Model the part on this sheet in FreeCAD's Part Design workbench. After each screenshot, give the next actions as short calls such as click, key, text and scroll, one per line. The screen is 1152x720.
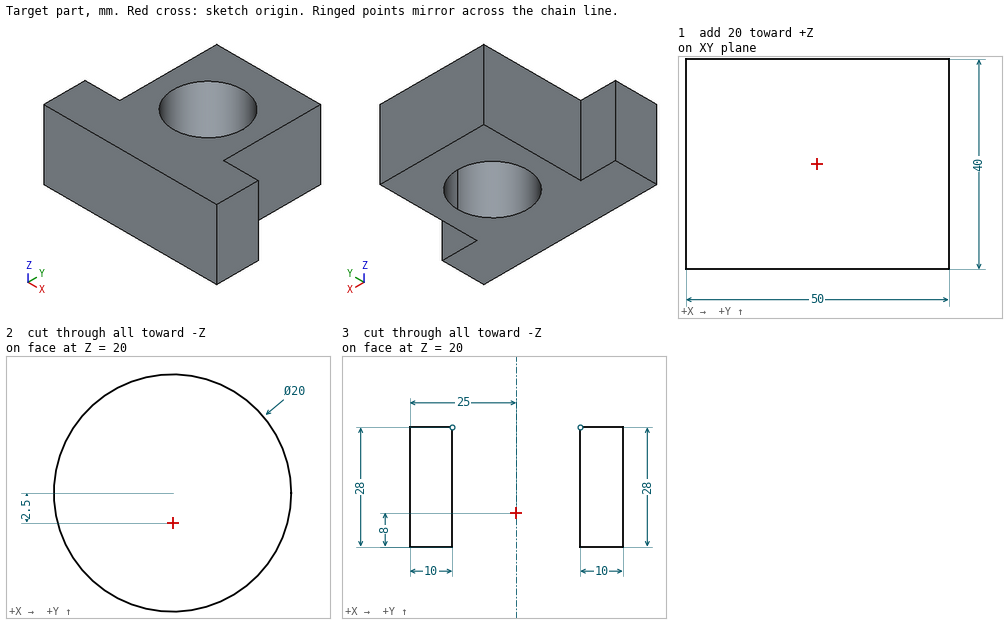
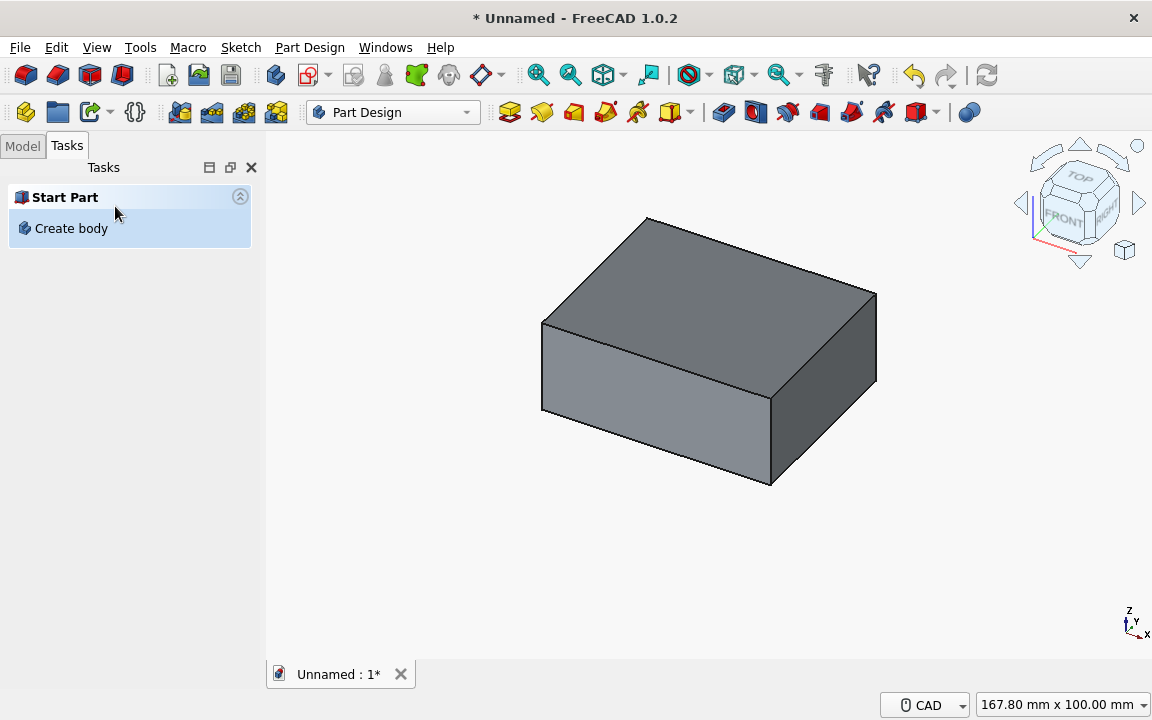
click(709, 307)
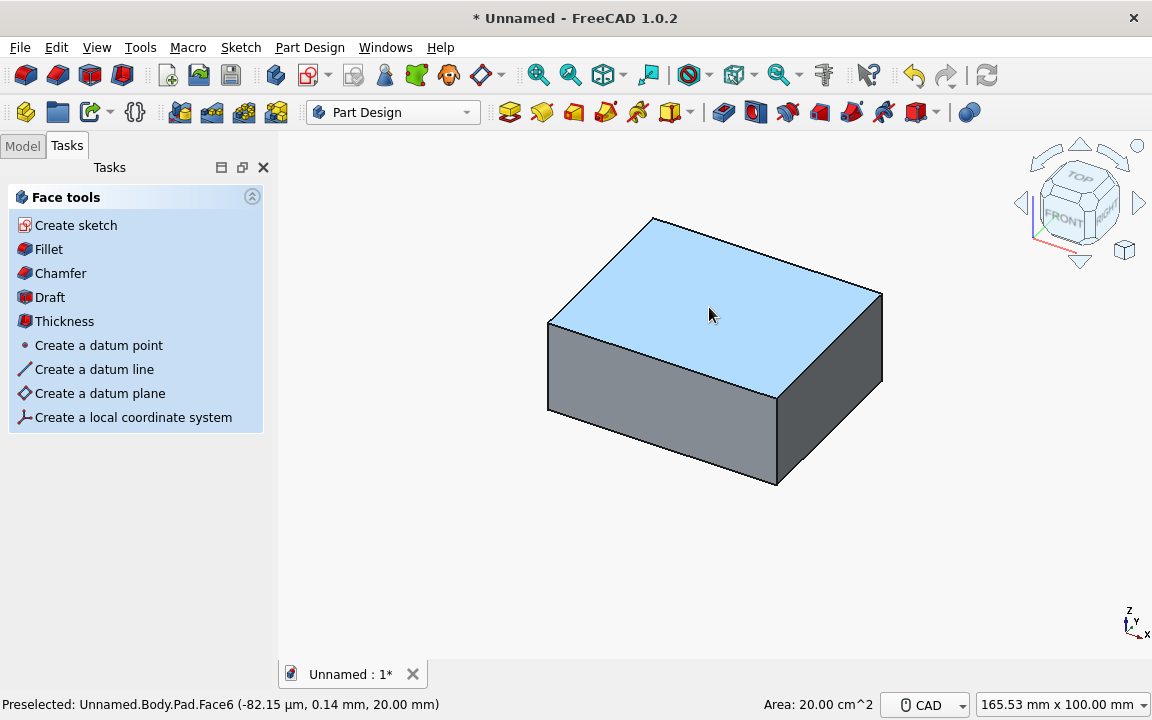
click(308, 76)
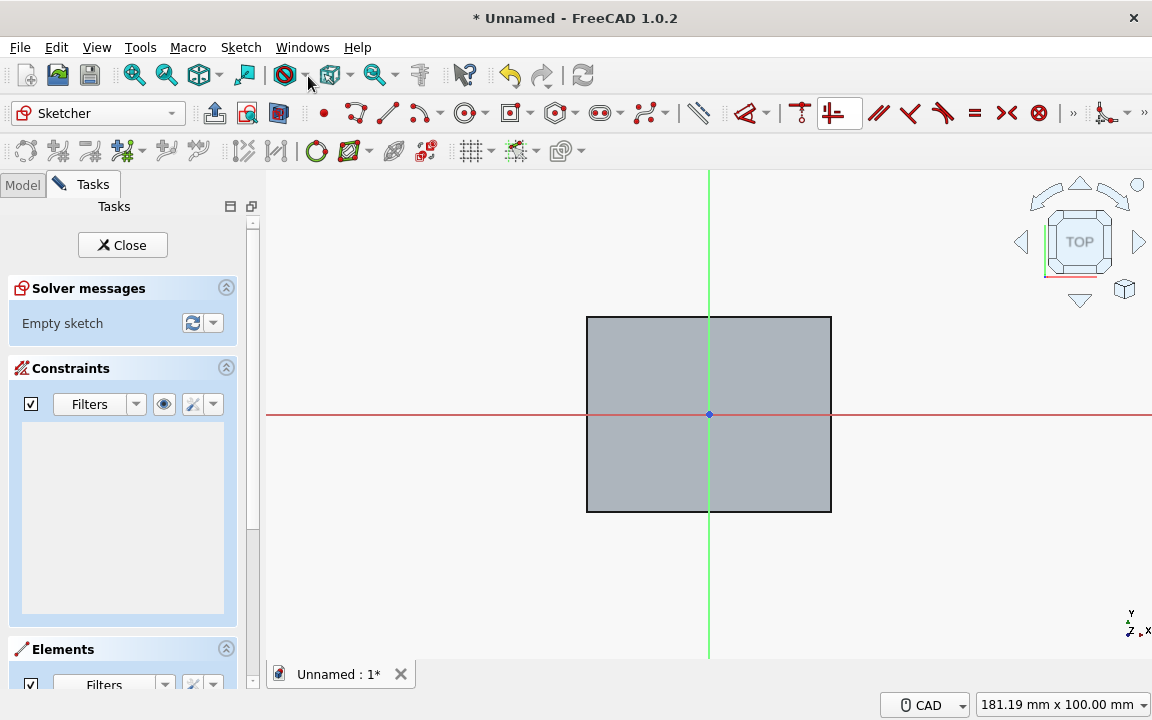
scroll(739, 397, up, 6)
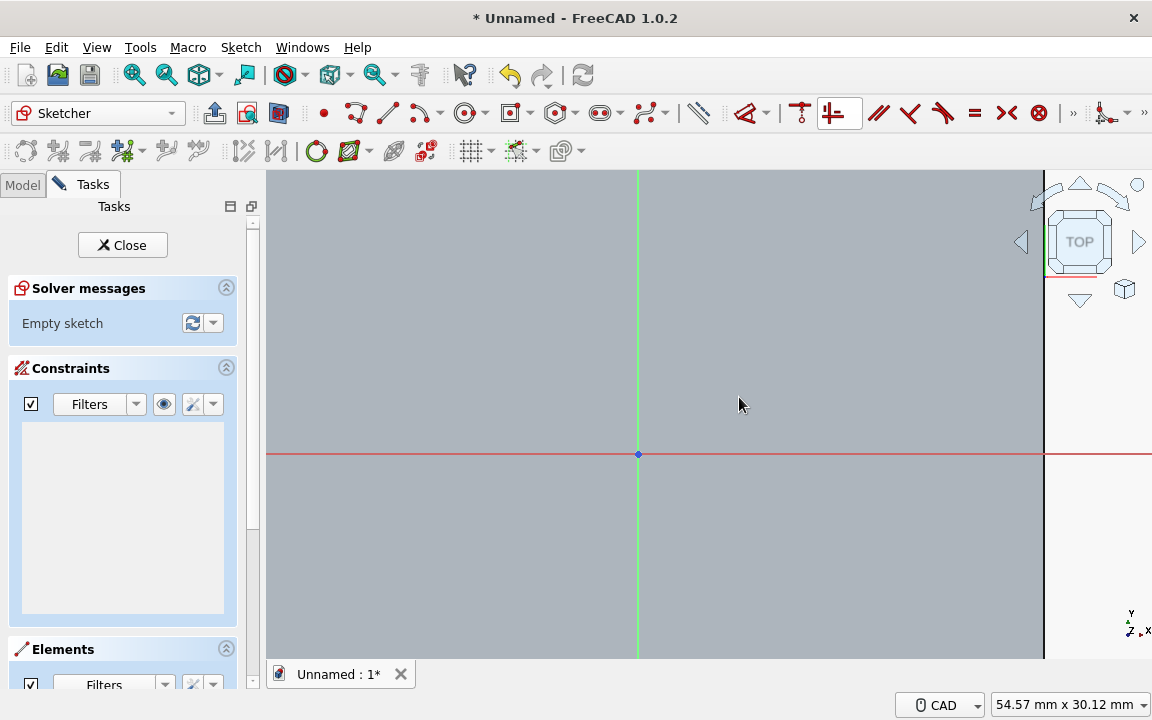
click(466, 114)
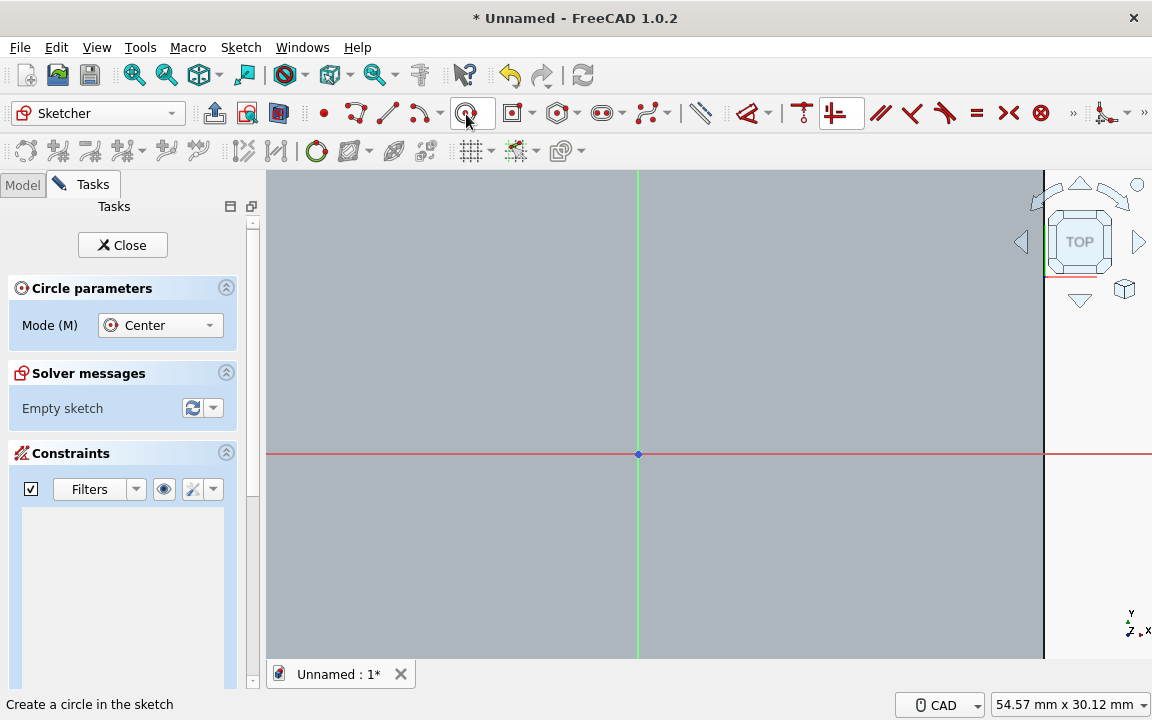
click(638, 413)
move(753, 299)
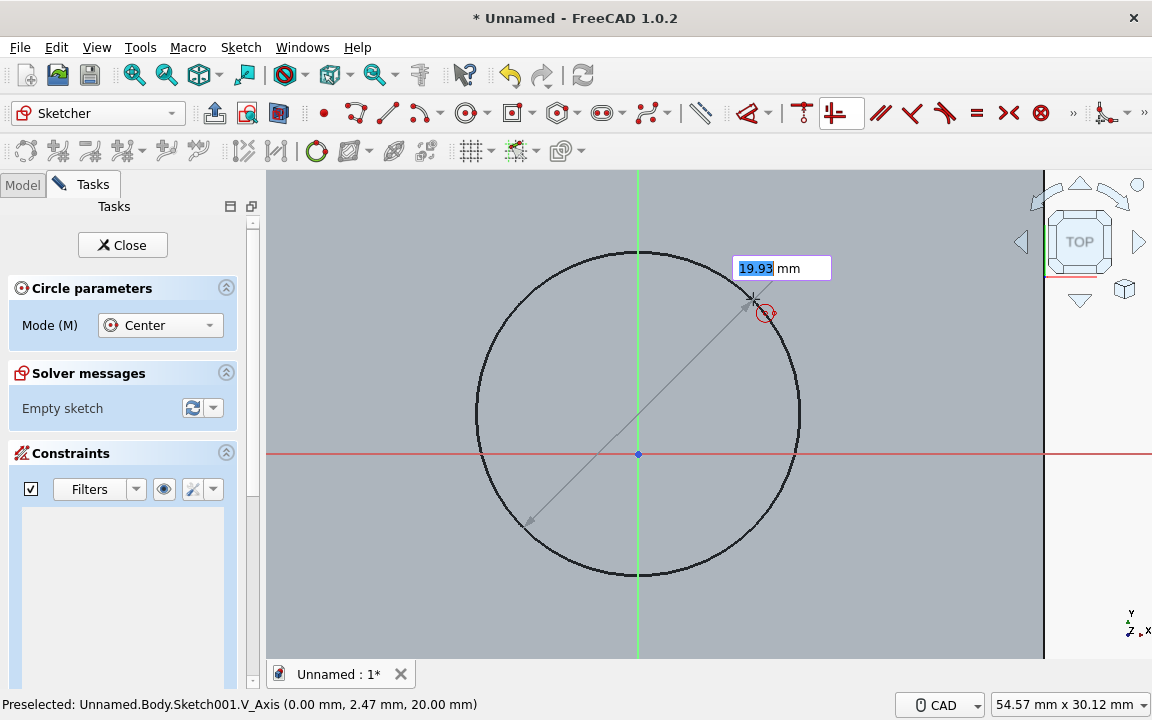
text(20)
key(Return)
key(Escape)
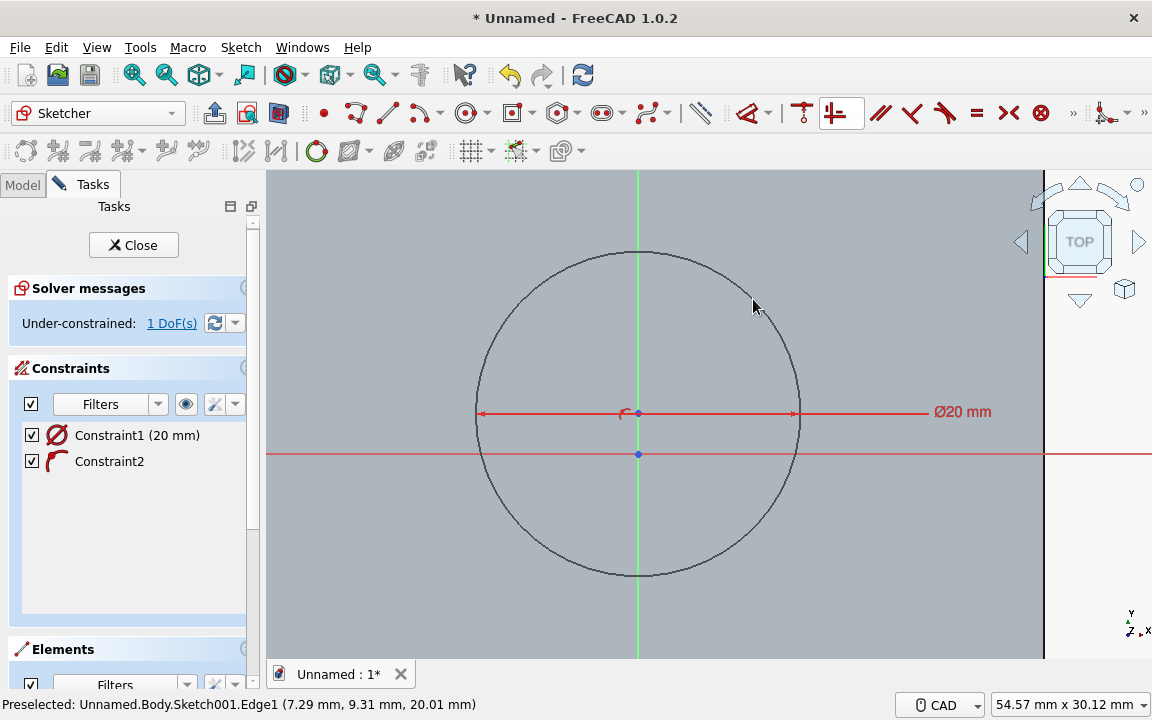
click(638, 414)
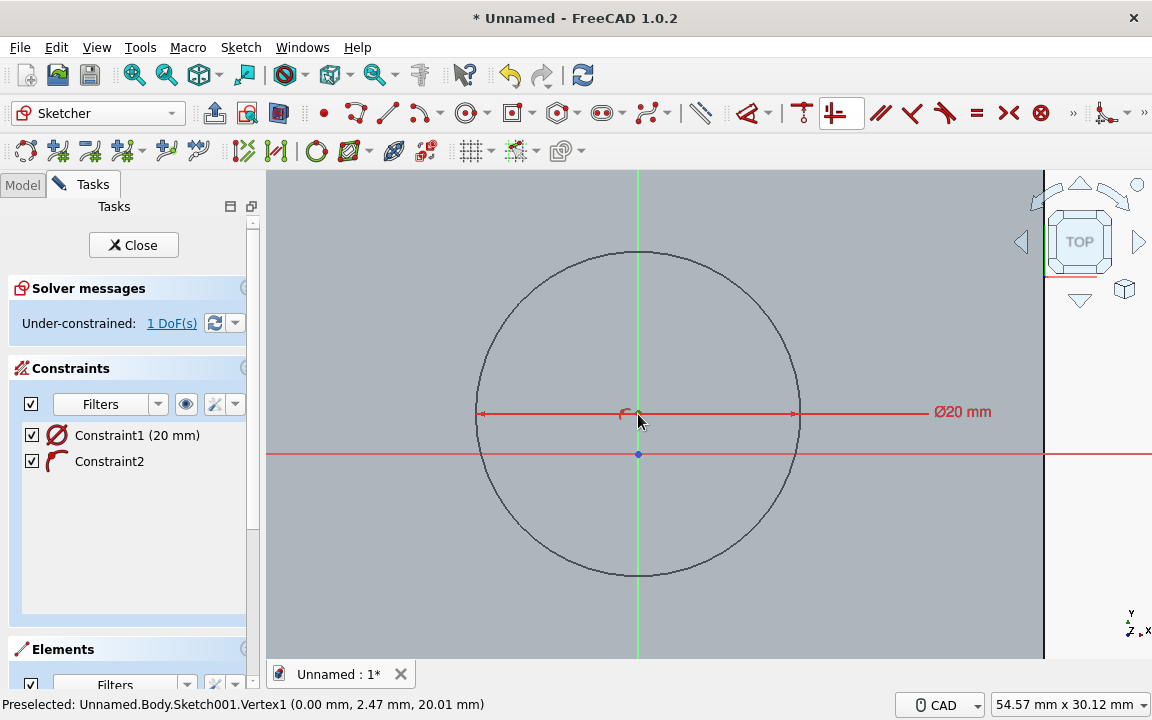
key(i)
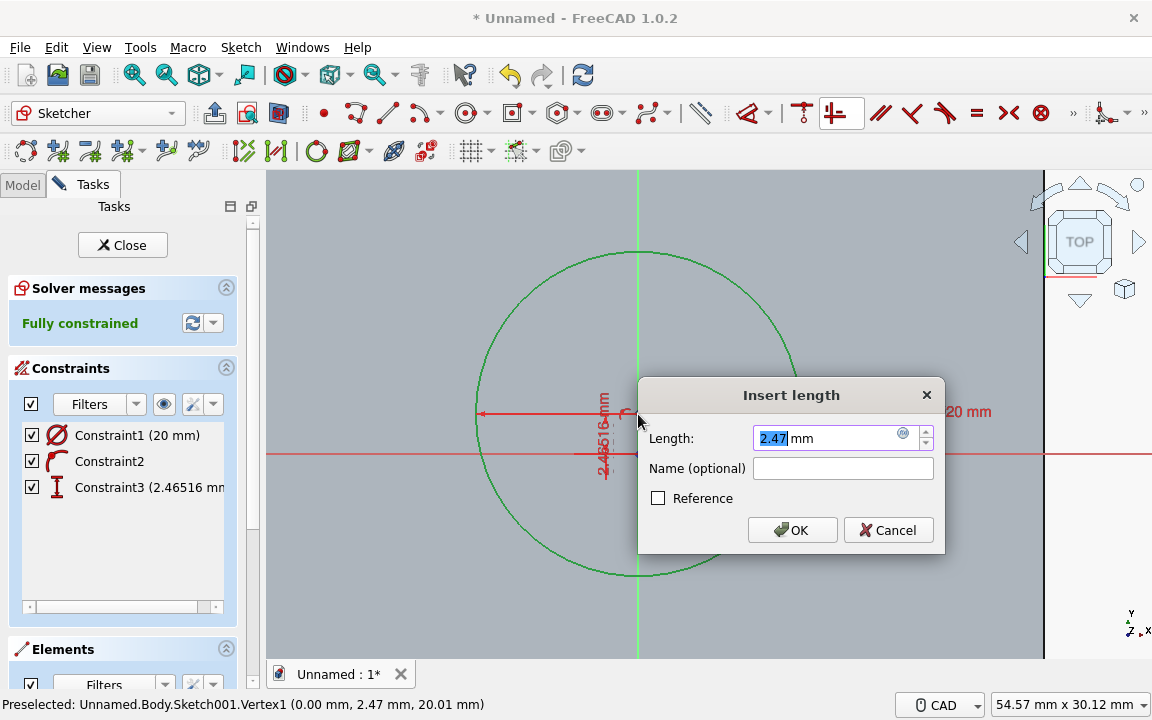
text(2.5)
key(Return)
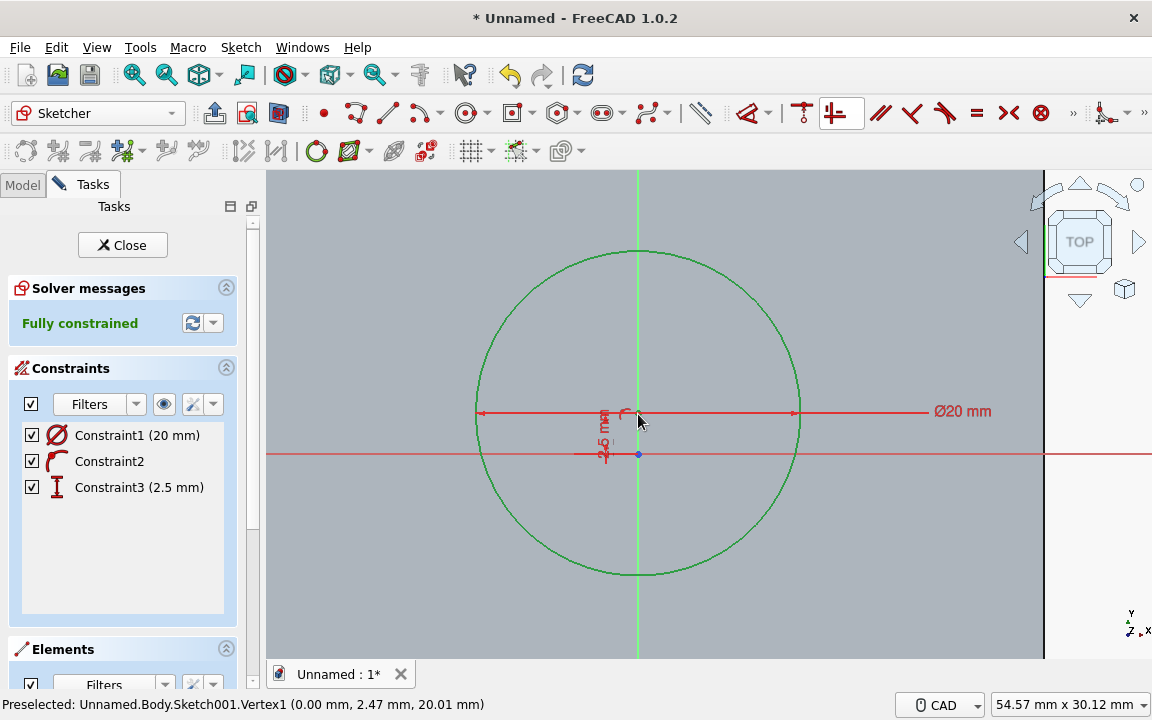
click(123, 245)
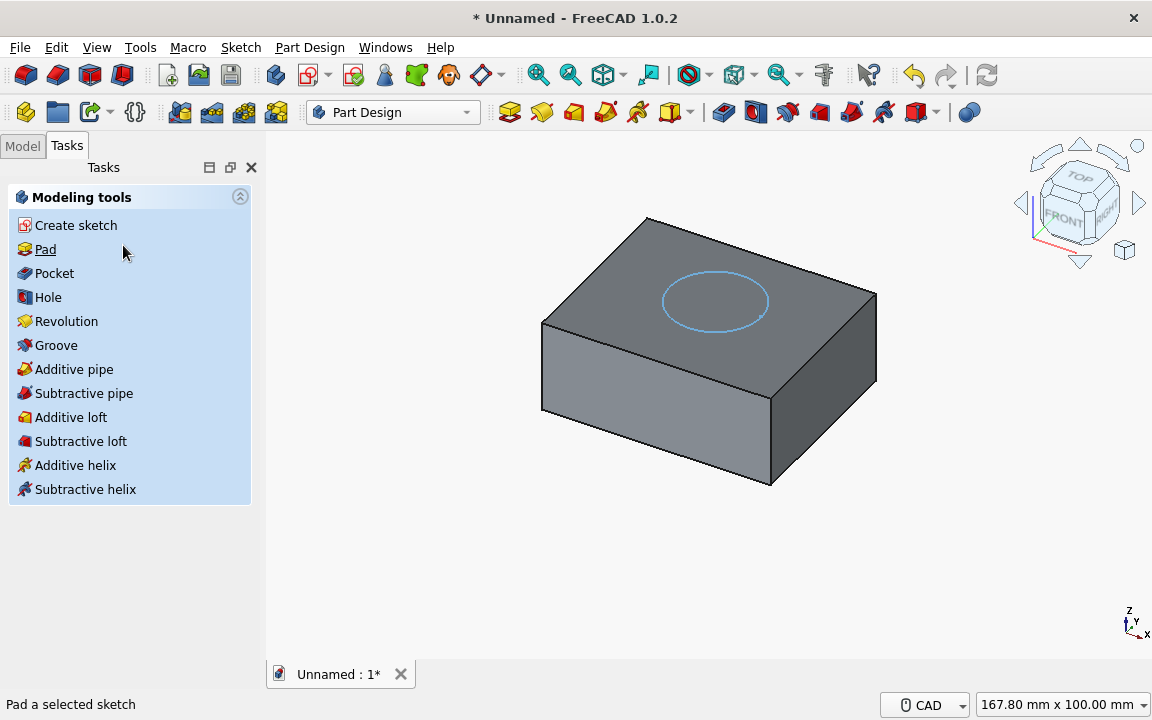
click(724, 112)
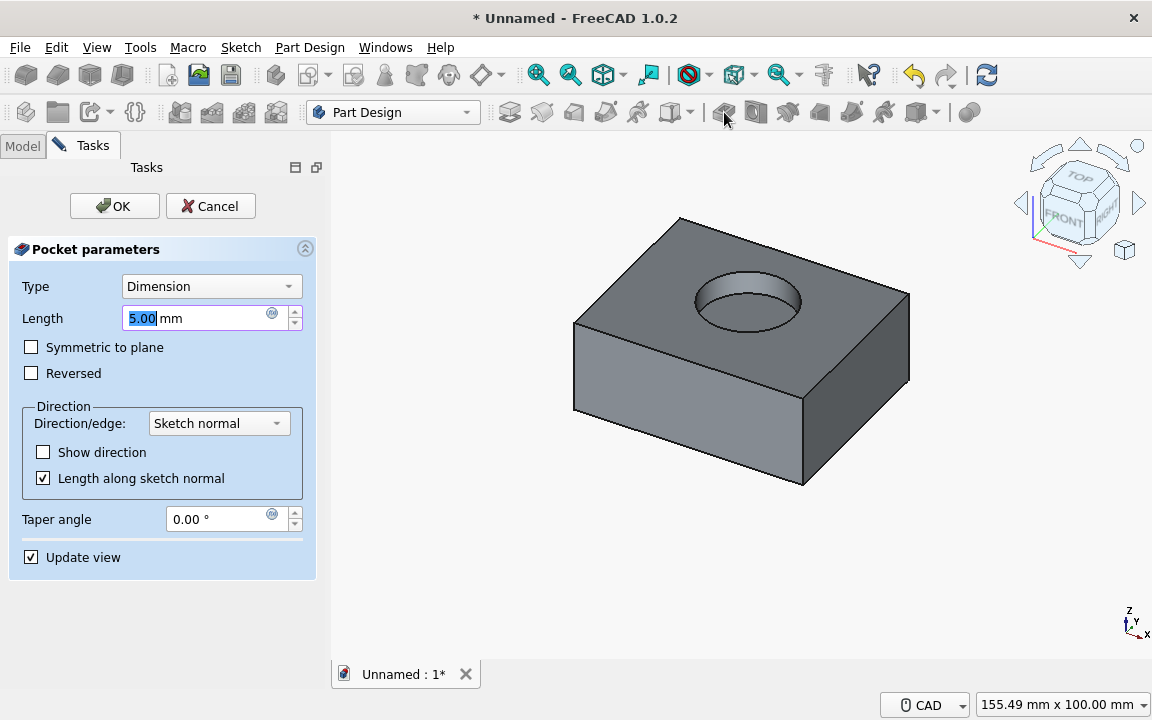
click(212, 286)